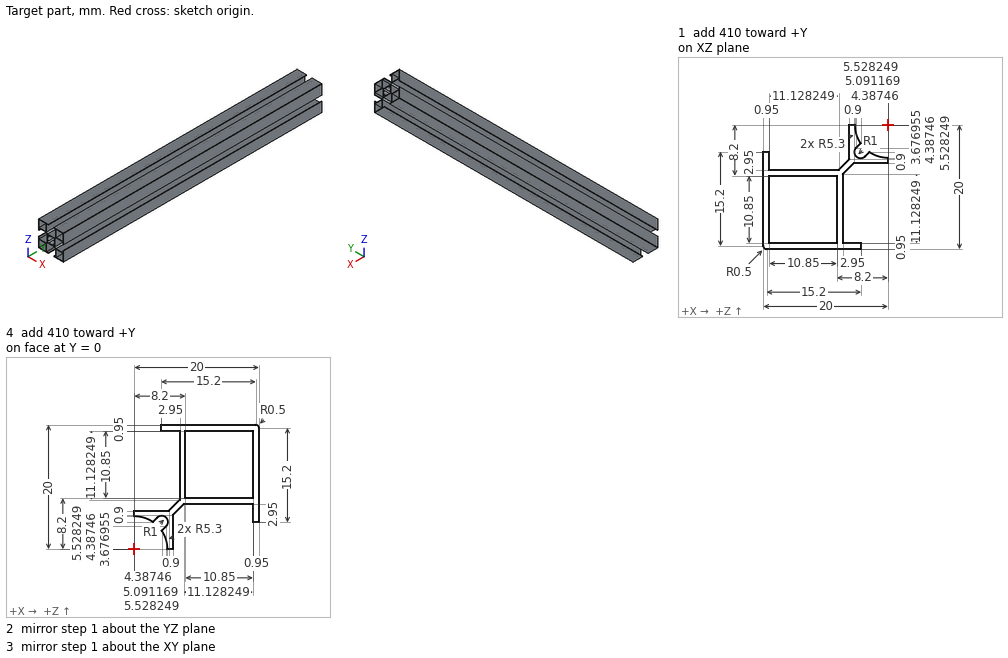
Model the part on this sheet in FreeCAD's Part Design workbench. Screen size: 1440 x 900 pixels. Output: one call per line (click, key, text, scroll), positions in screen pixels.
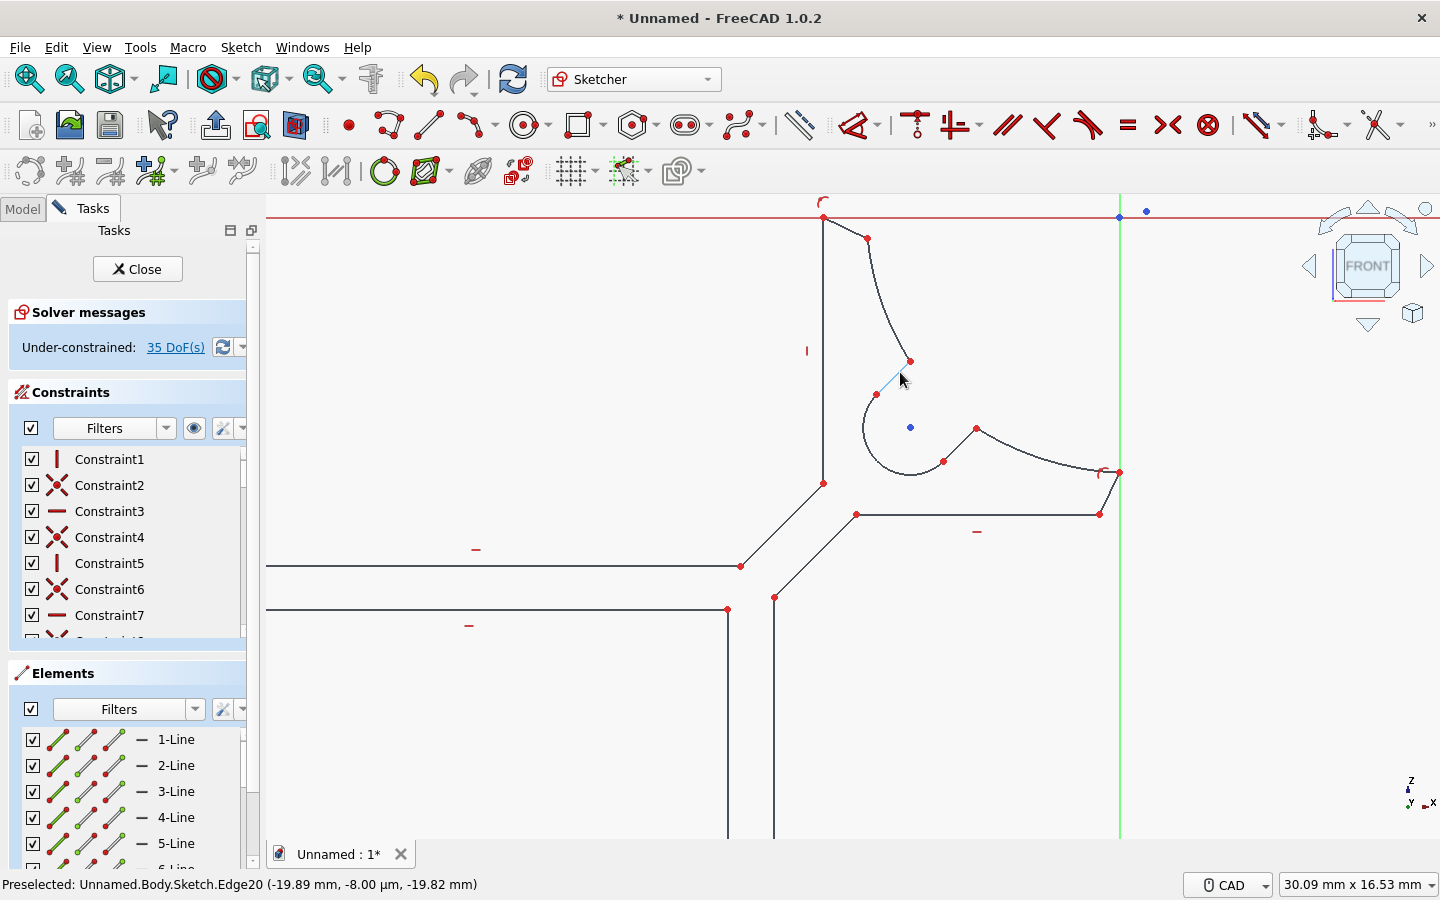
click(900, 371)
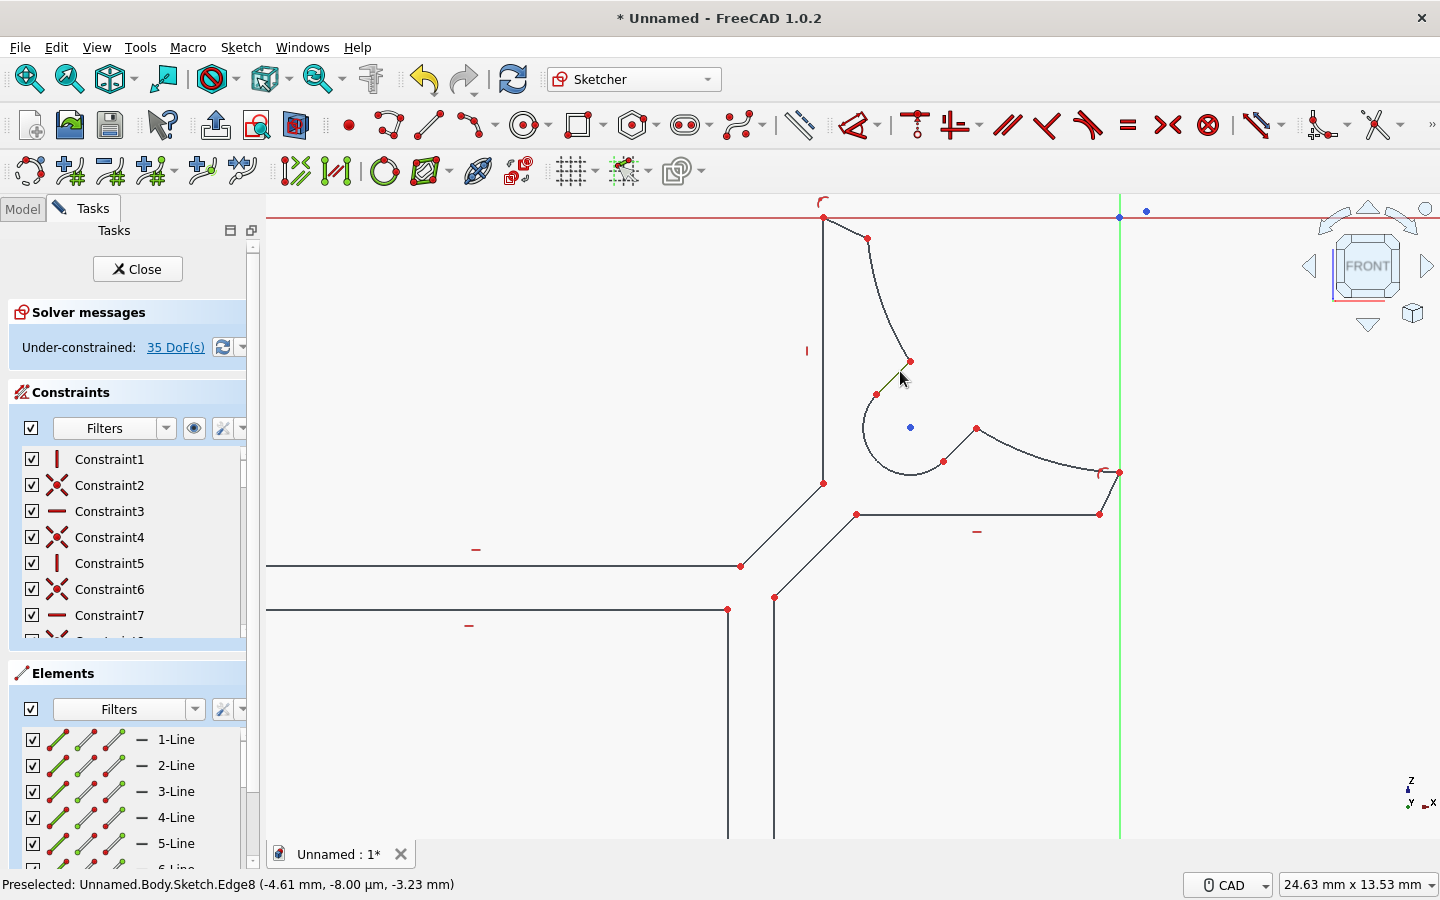
click(864, 435)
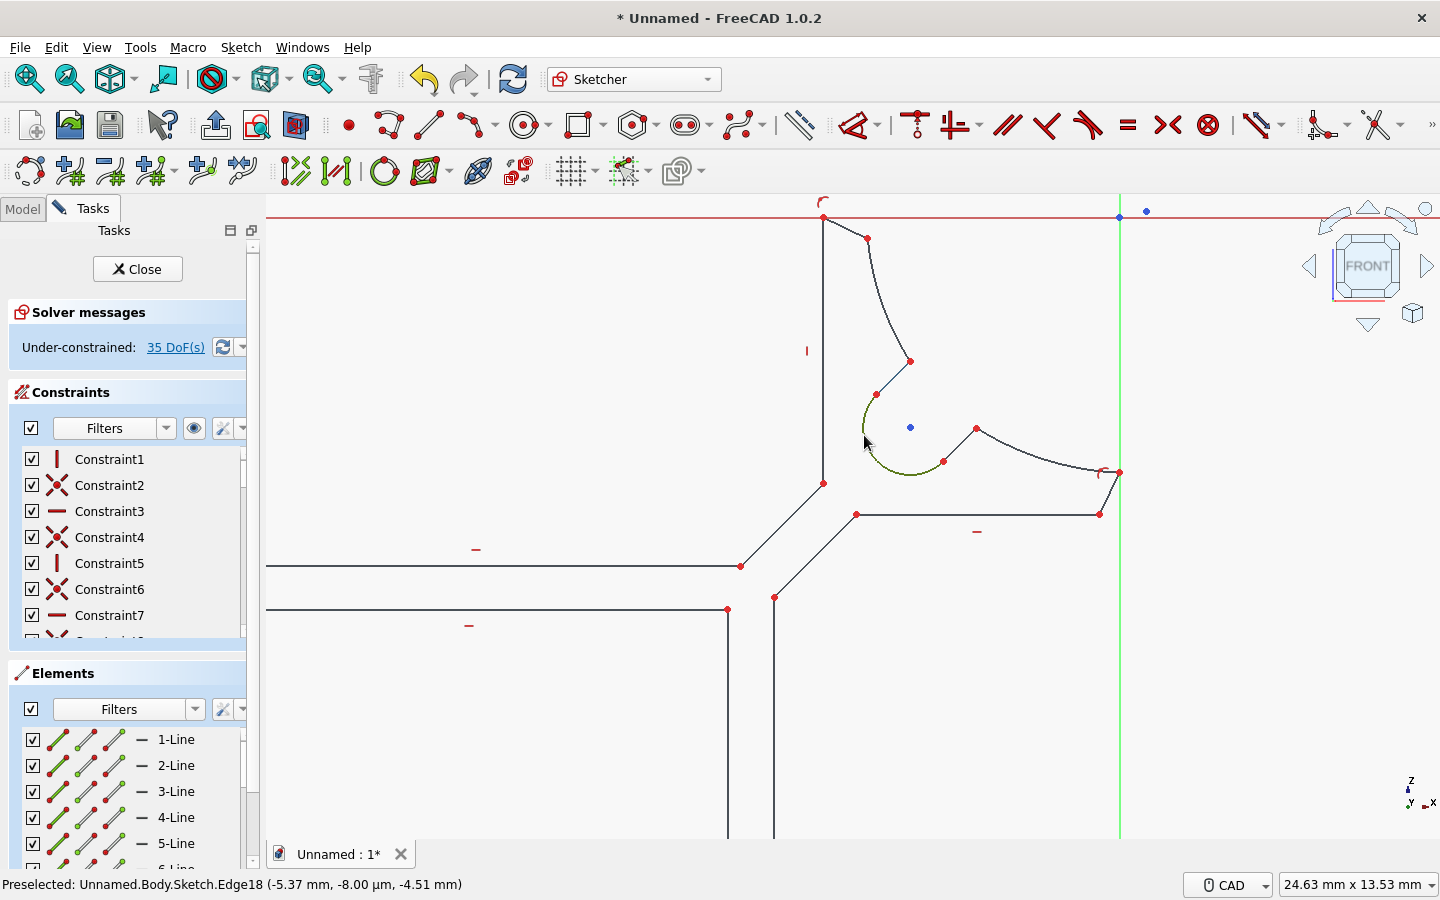
click(1088, 126)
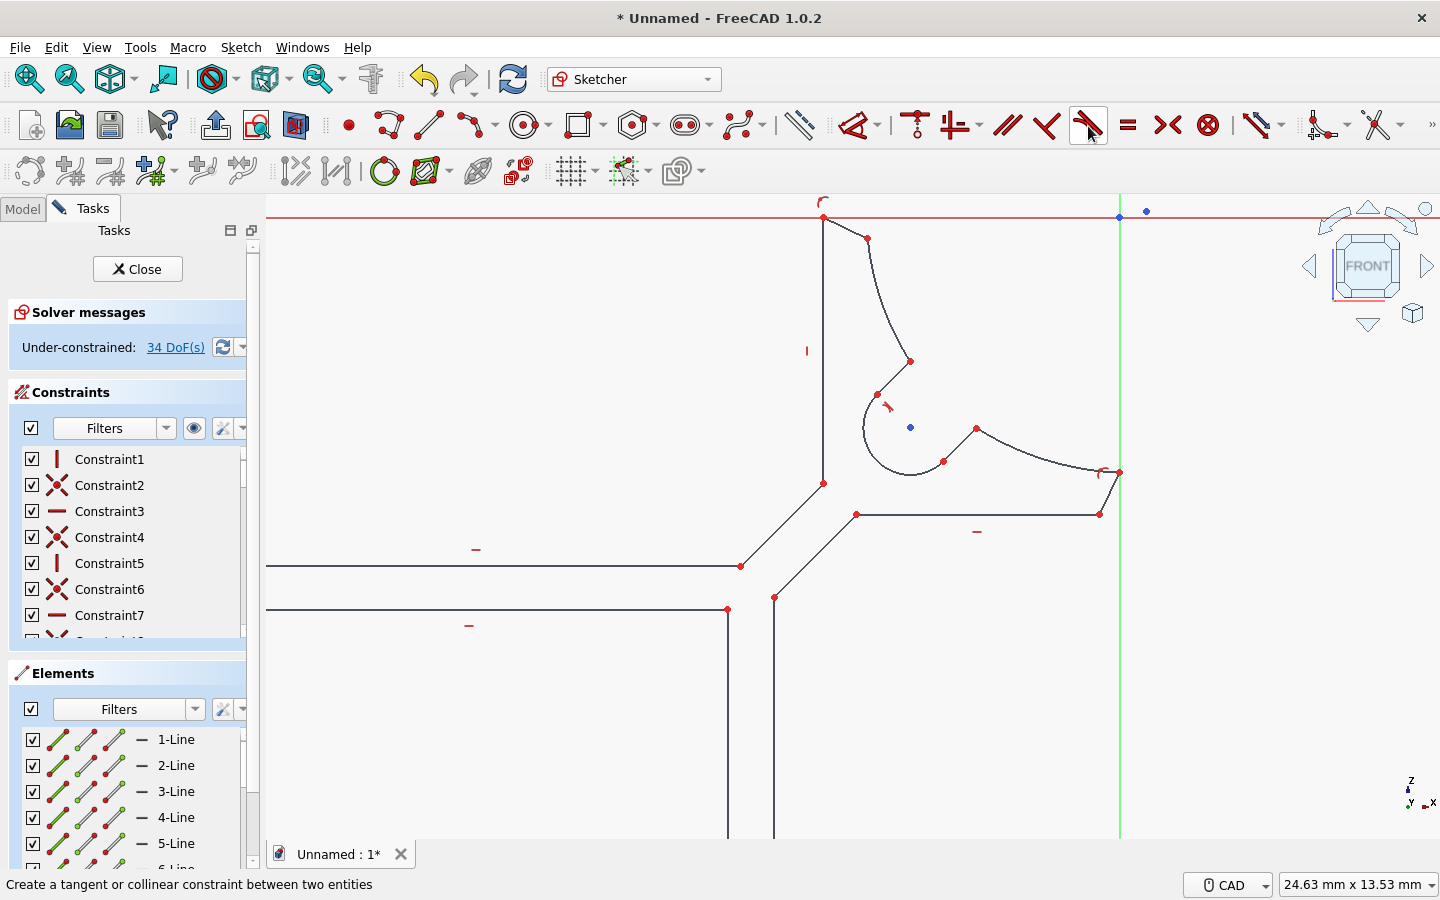
click(953, 451)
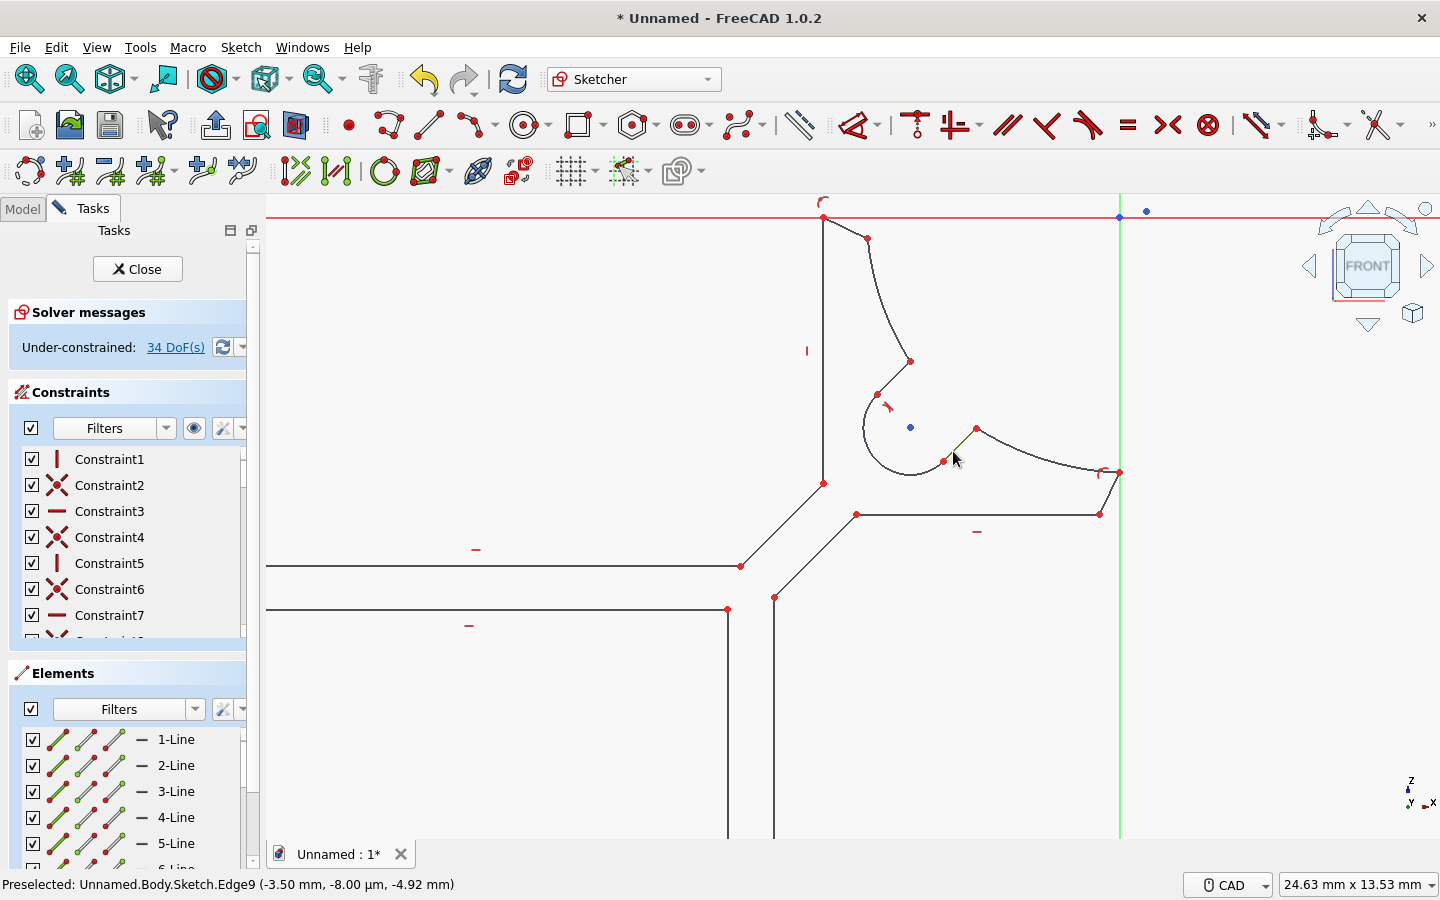
click(864, 435)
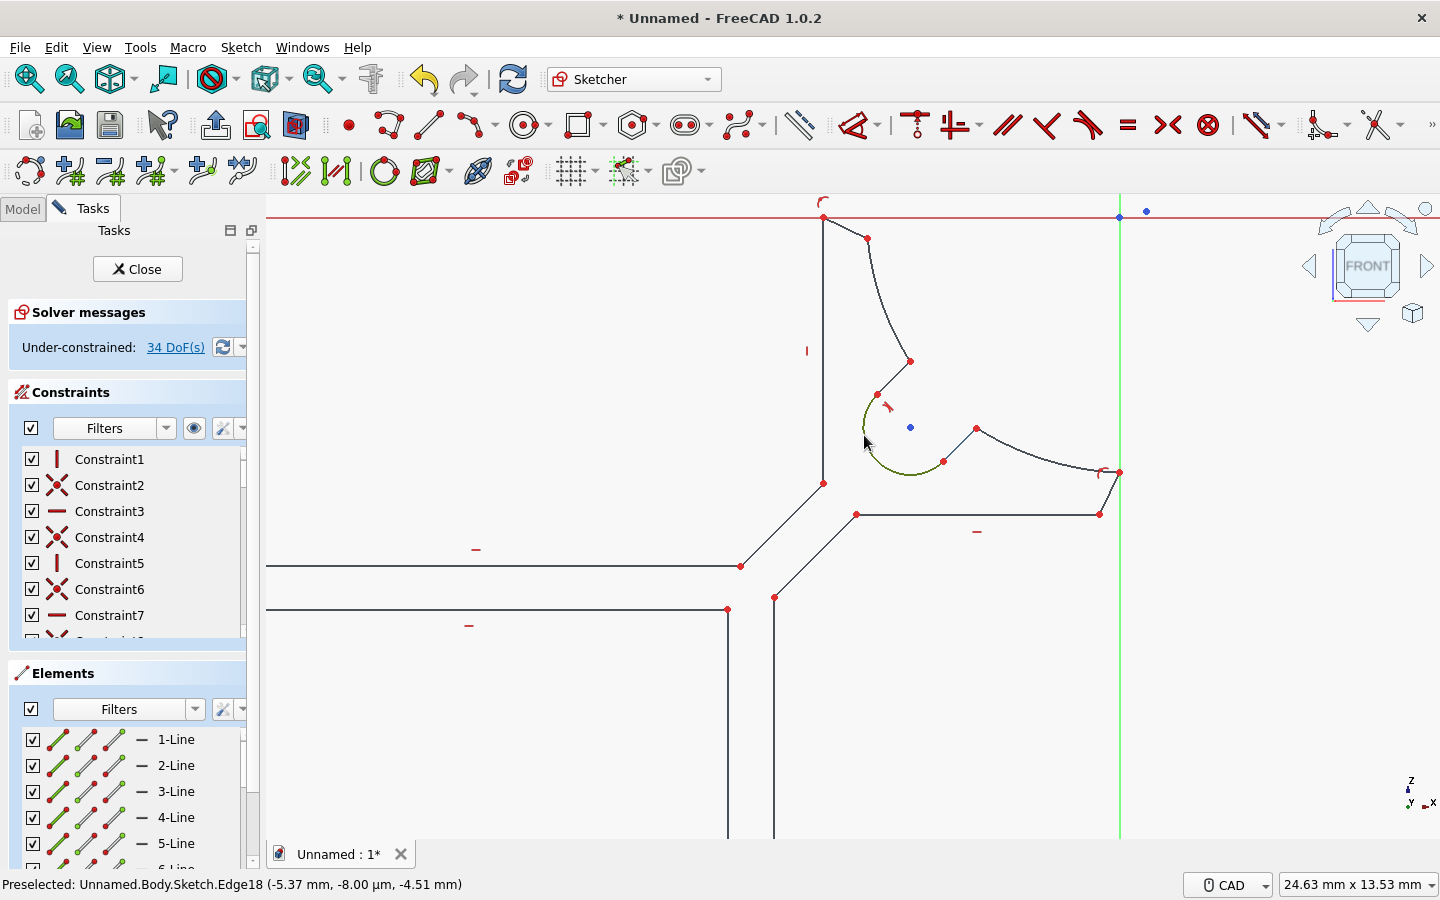
key(t)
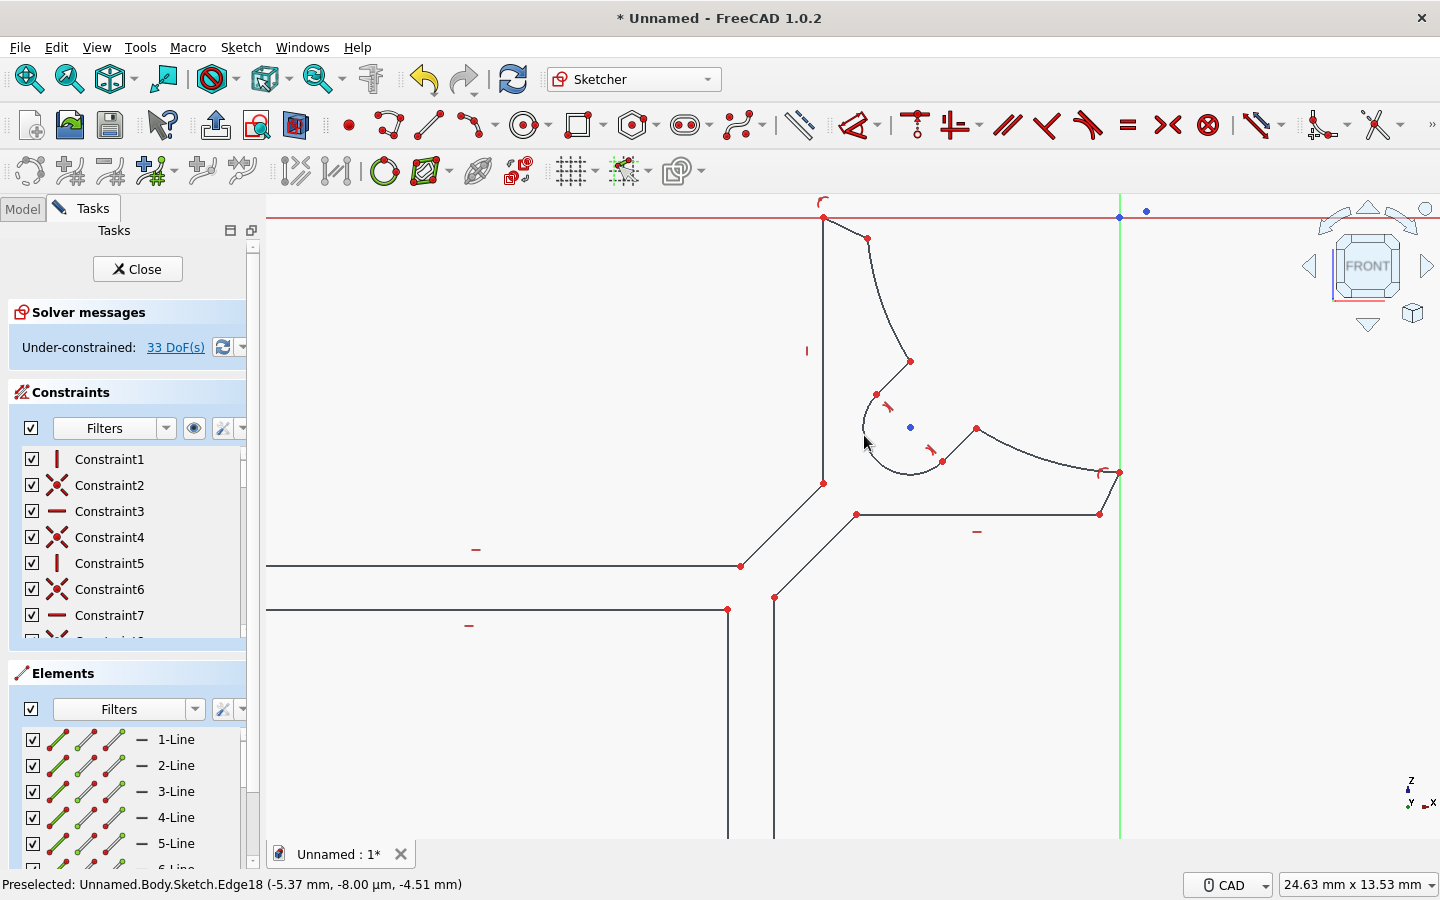
scroll(900, 372, down, 4)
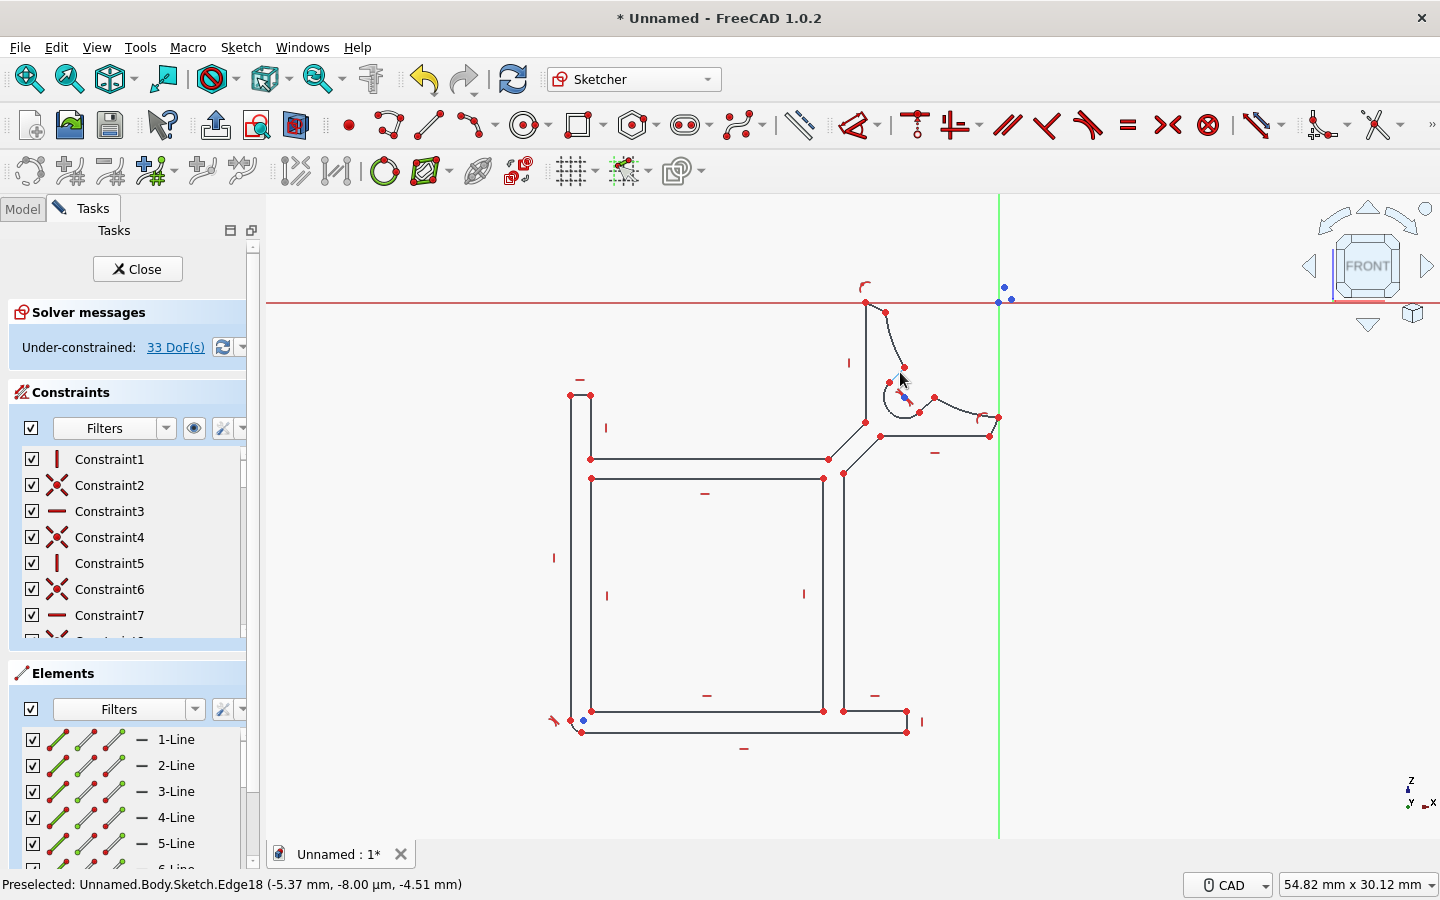
click(809, 733)